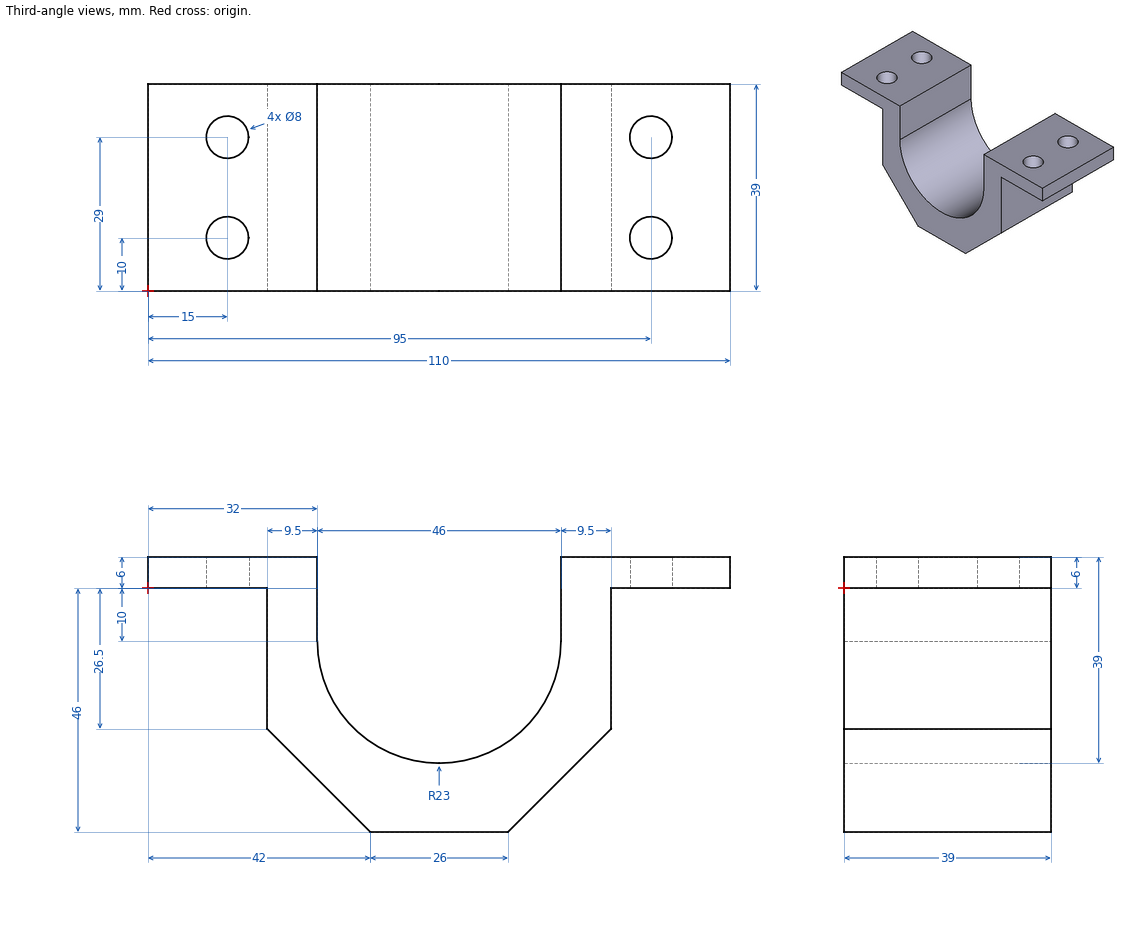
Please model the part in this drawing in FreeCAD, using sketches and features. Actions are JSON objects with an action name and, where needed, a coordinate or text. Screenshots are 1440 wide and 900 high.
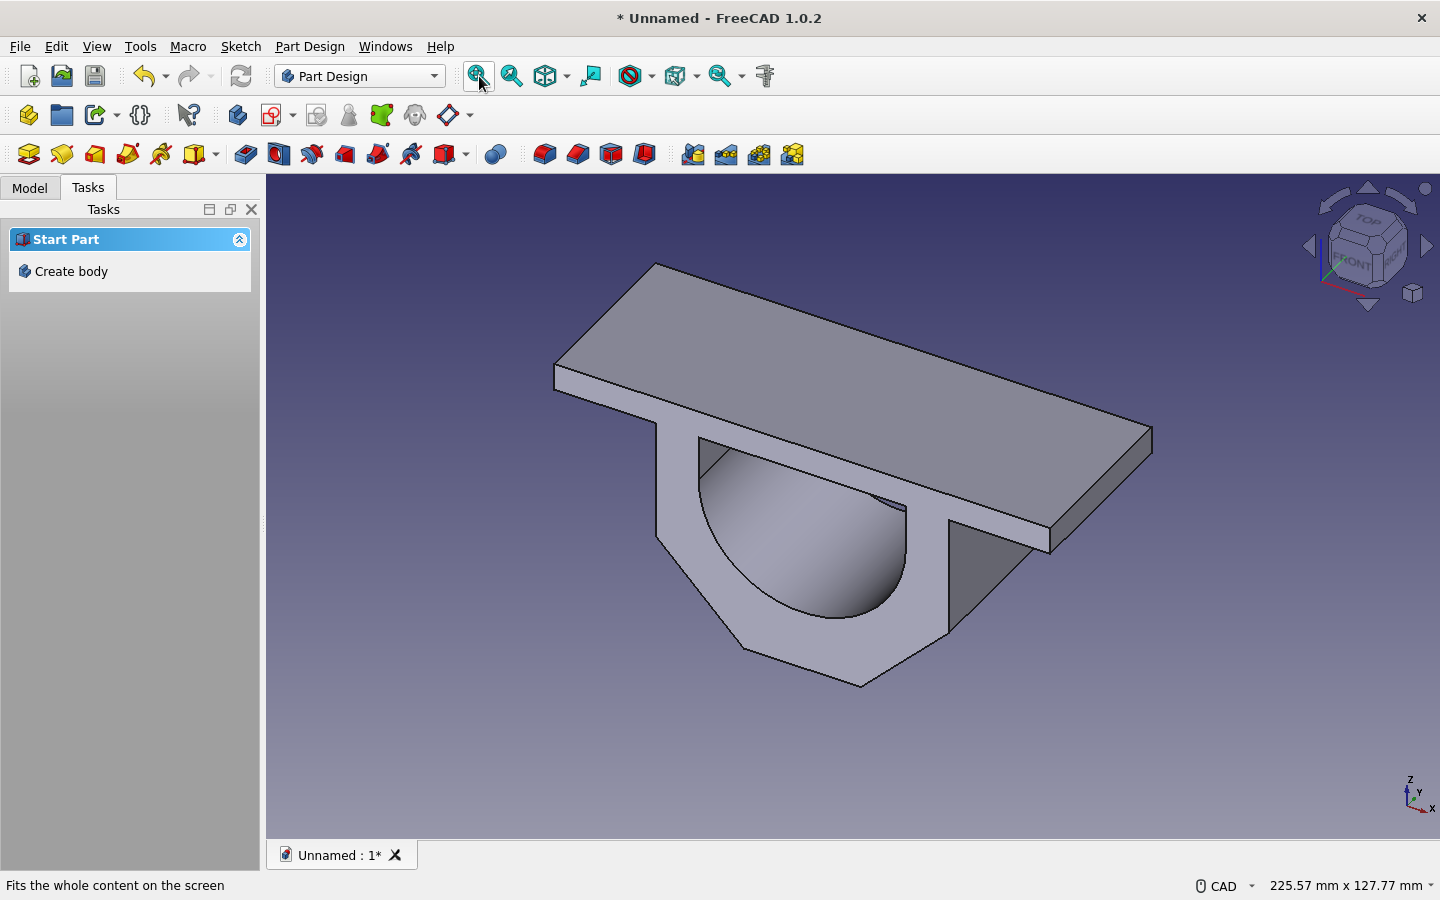
{"action": "left_click", "coordinate": [270, 116]}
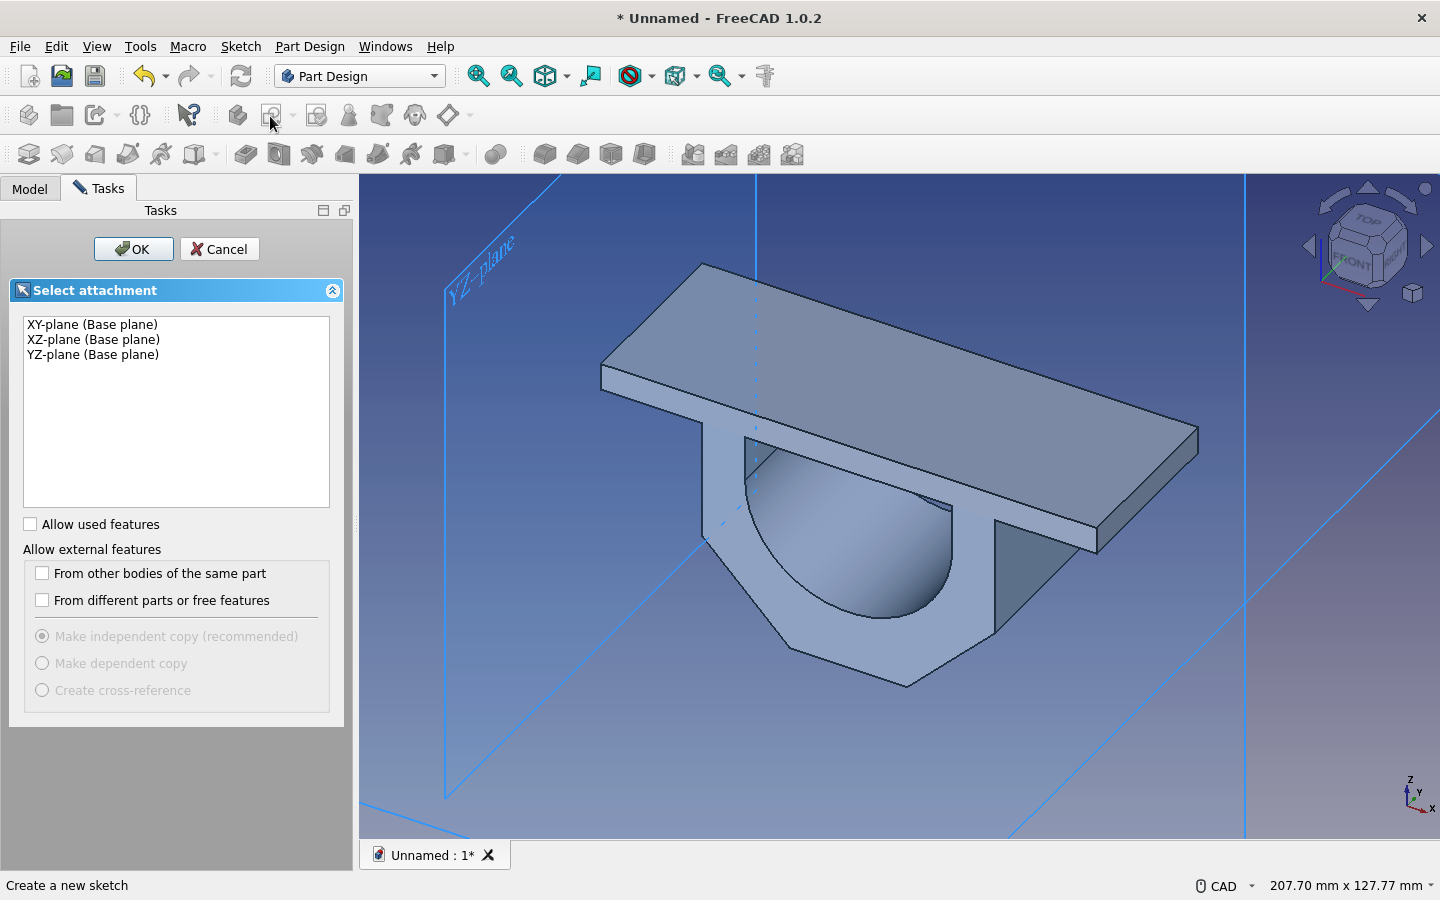
{"action": "left_click", "coordinate": [84, 340]}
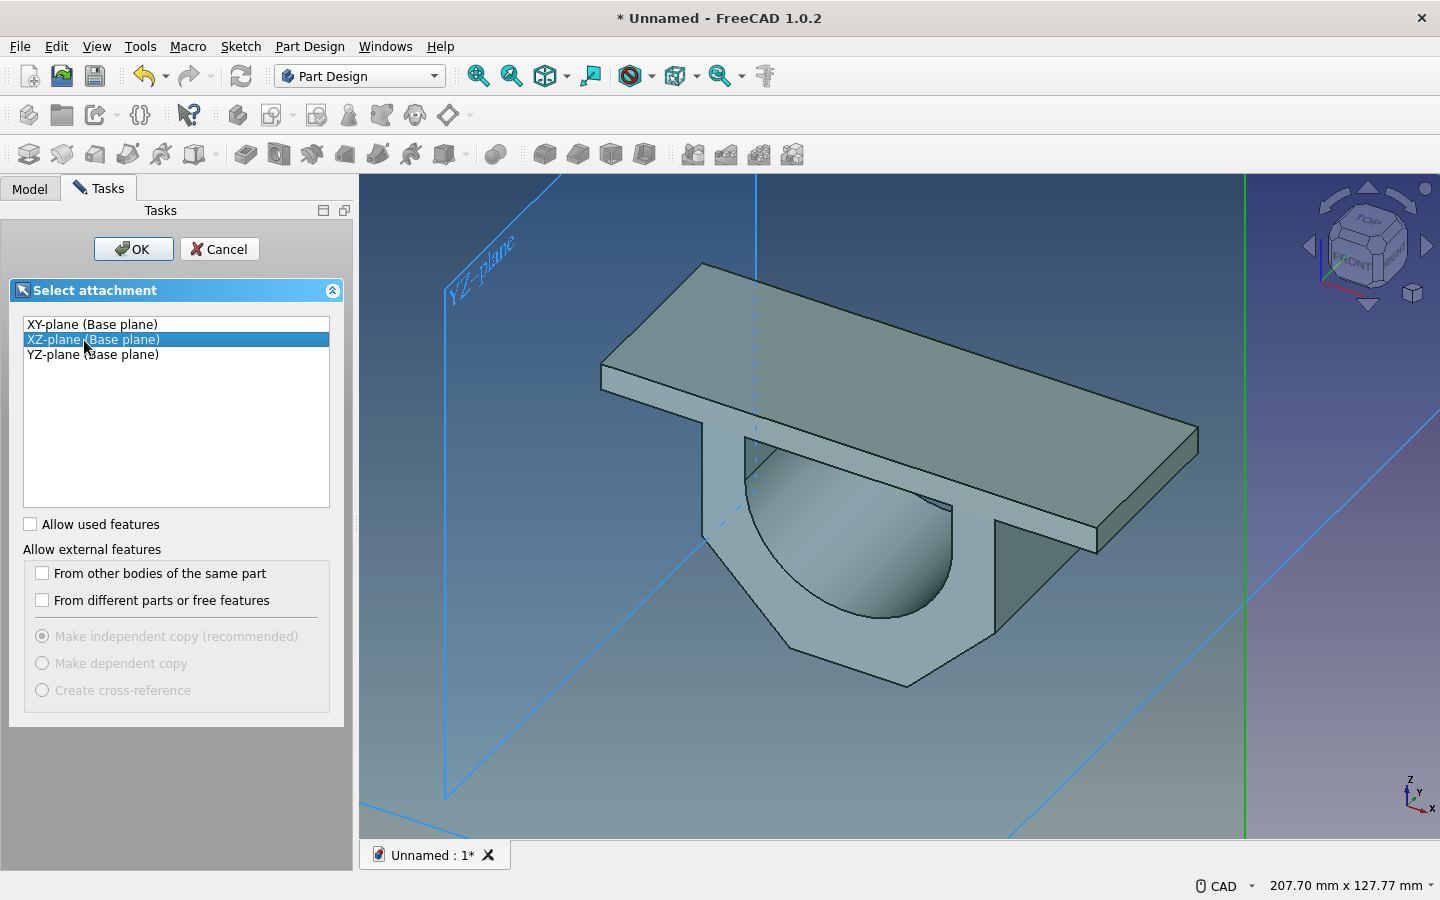
{"action": "left_click", "coordinate": [134, 249]}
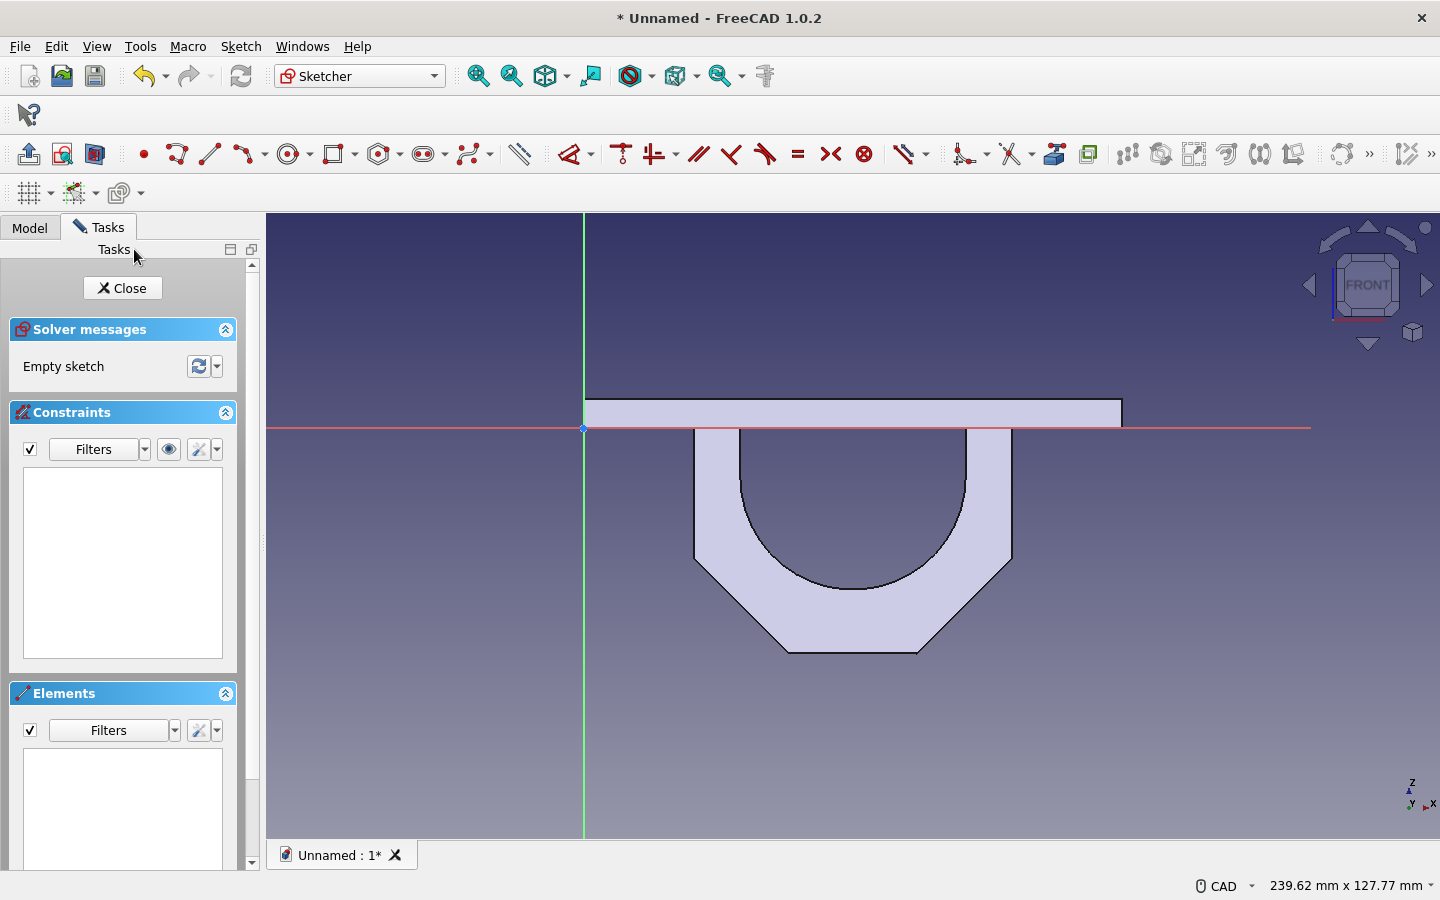
{"action": "scroll", "coordinate": [763, 276], "scroll_direction": "up", "scroll_amount": 3}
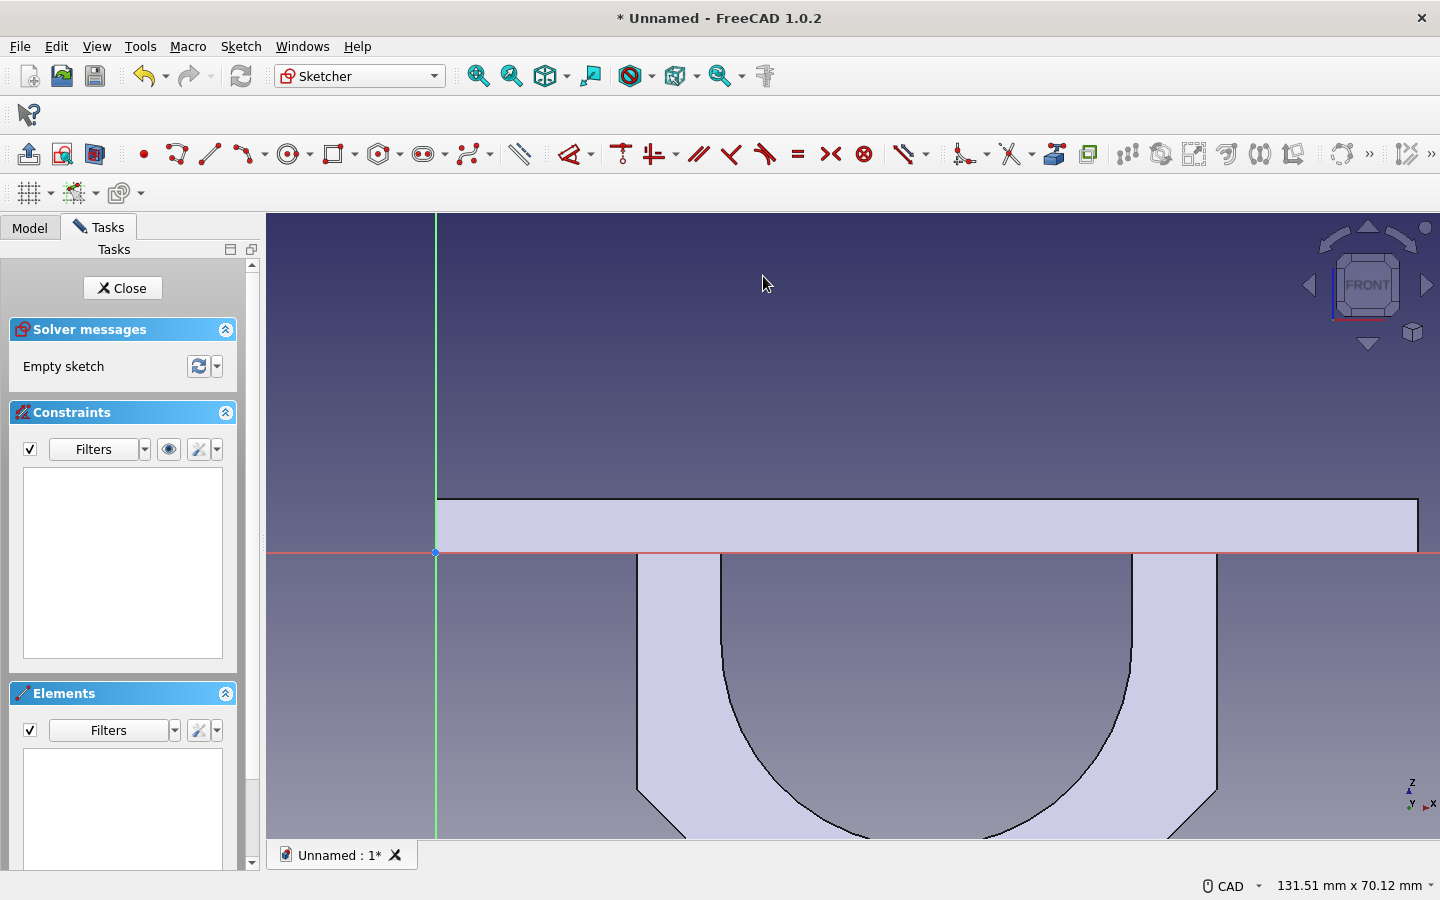
{"action": "key", "text": "g r"}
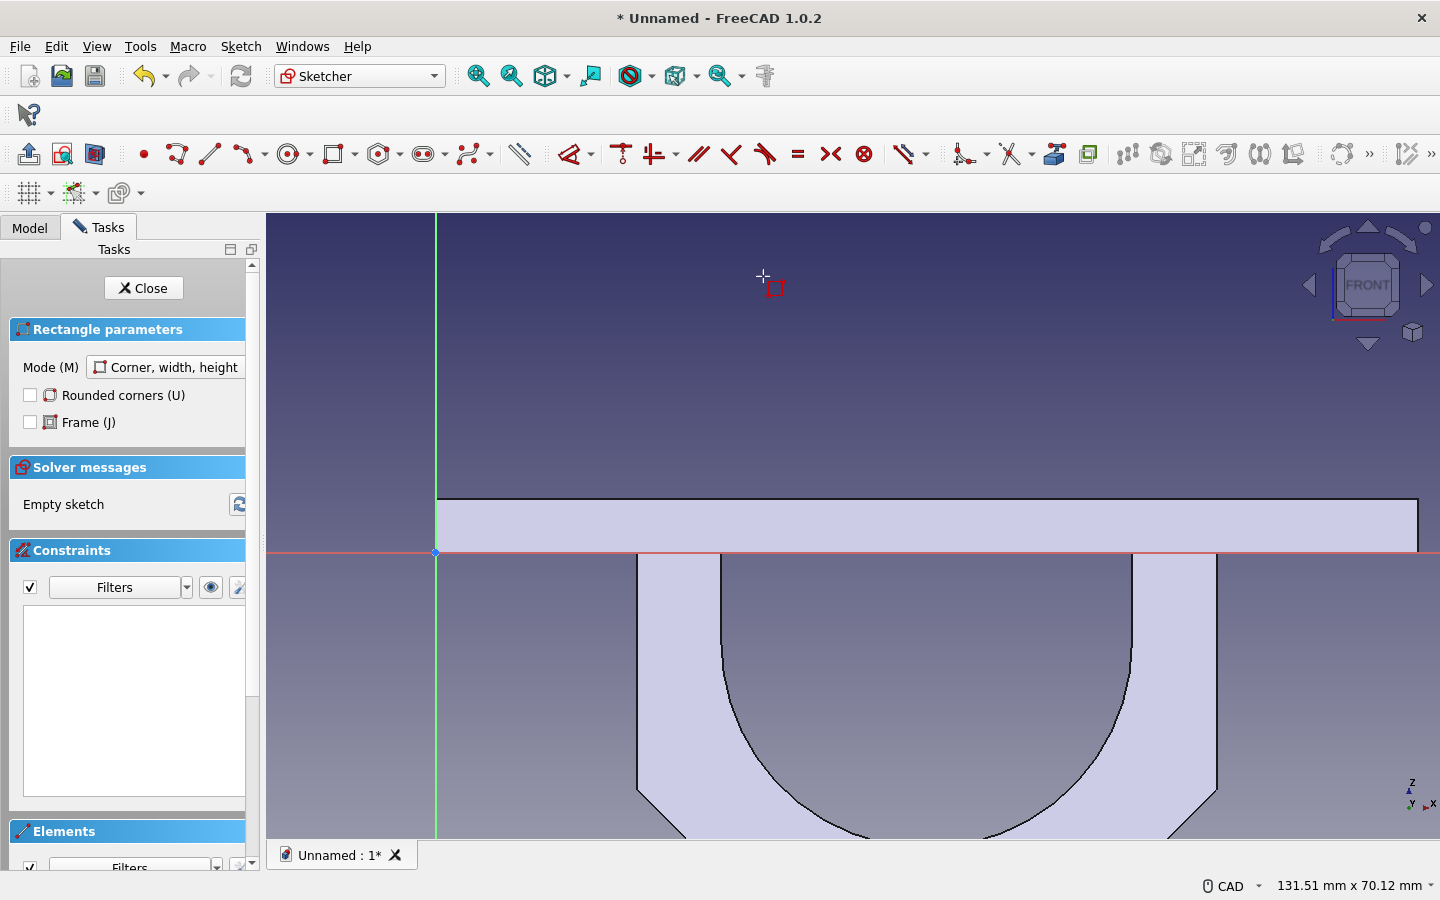
{"action": "left_click", "coordinate": [721, 499]}
{"action": "left_click", "coordinate": [1132, 553]}
{"action": "key", "text": "Escape"}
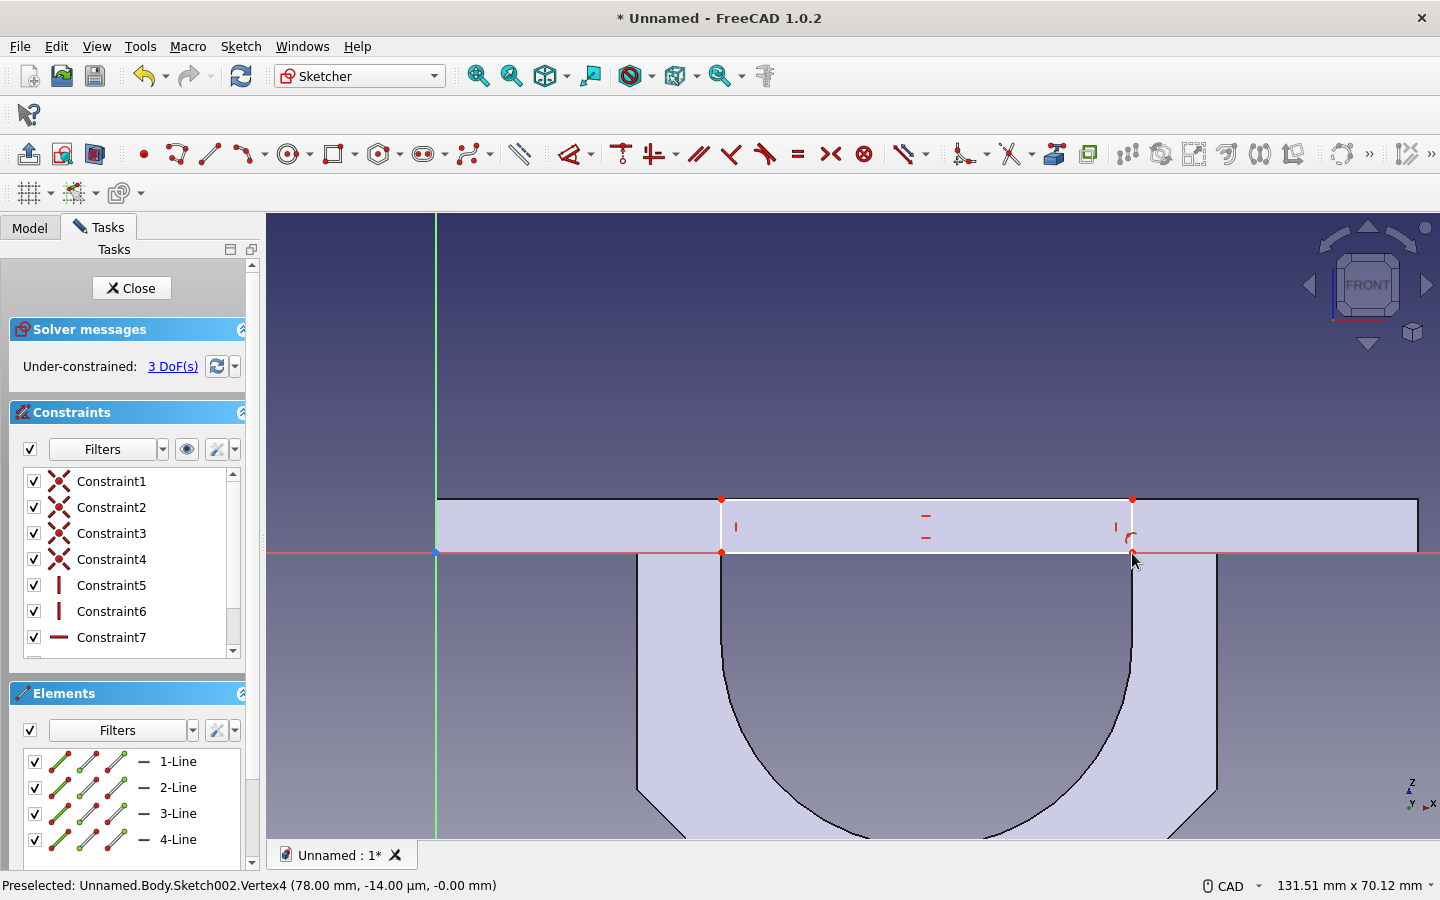
{"action": "key", "text": "d"}